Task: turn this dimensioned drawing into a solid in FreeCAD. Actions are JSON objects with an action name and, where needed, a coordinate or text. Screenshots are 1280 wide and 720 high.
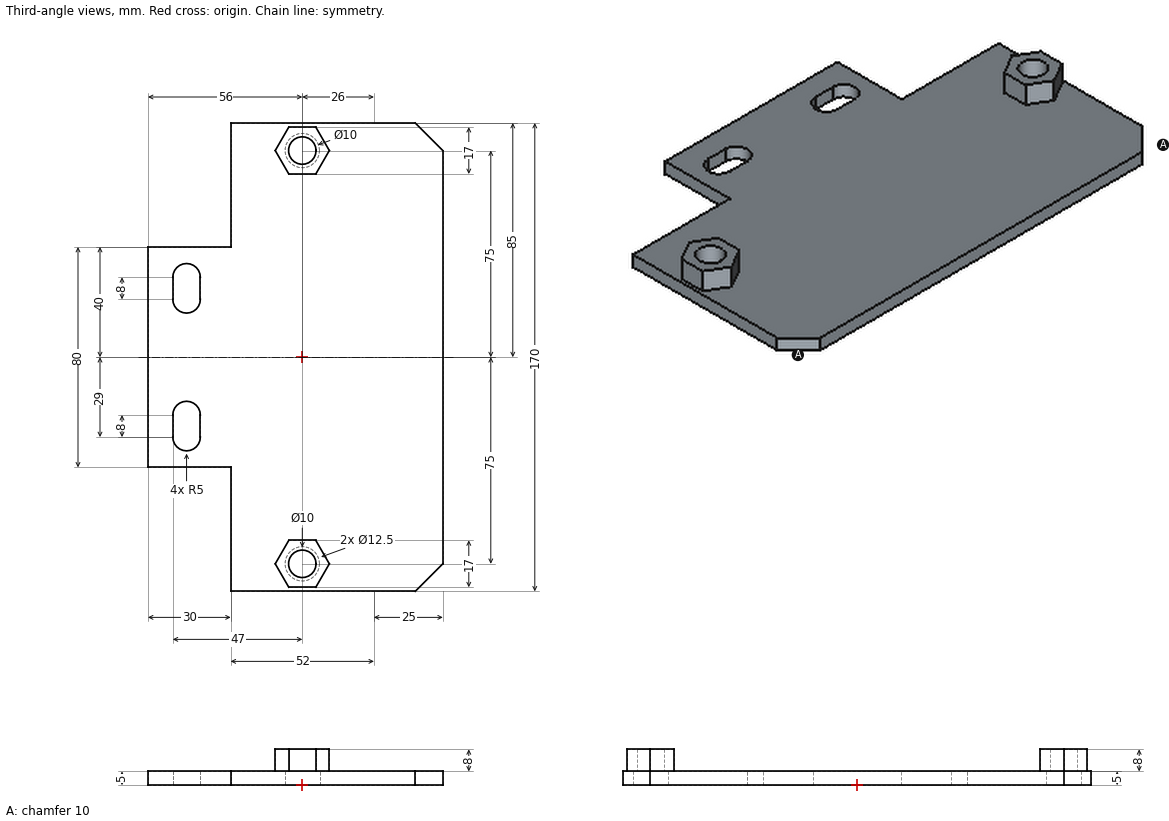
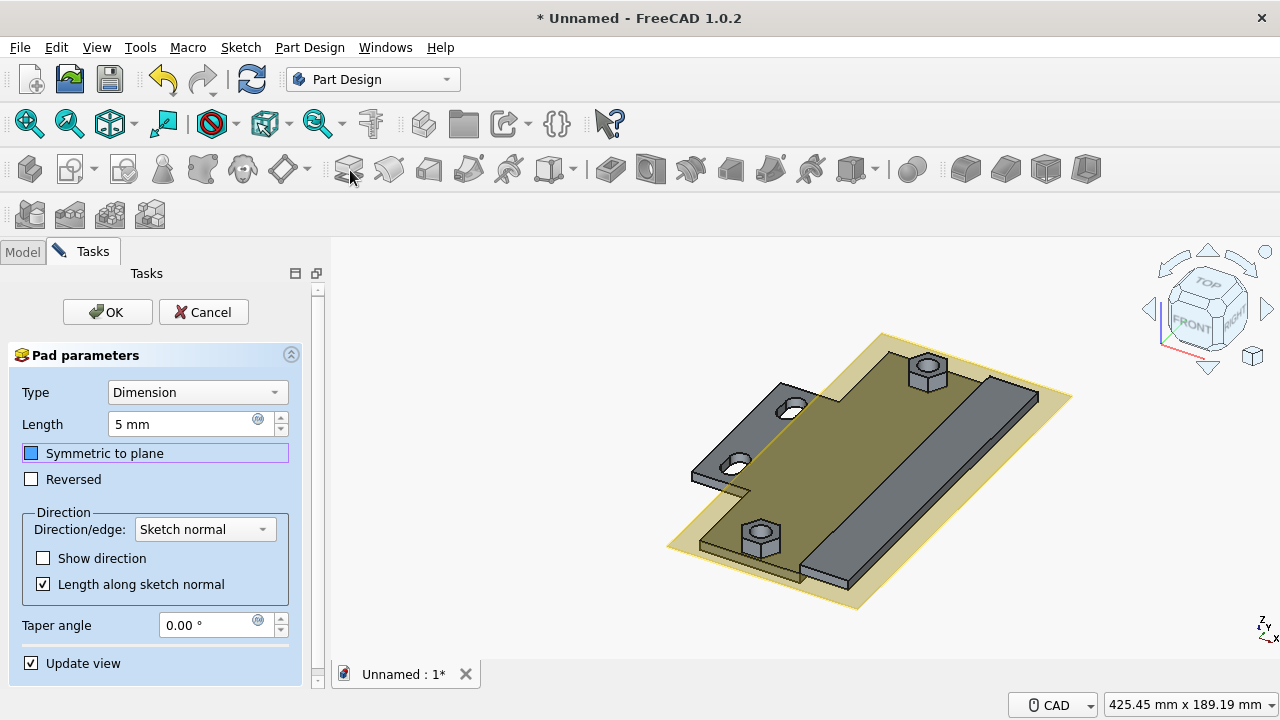
{"action": "left_click", "coordinate": [30, 479]}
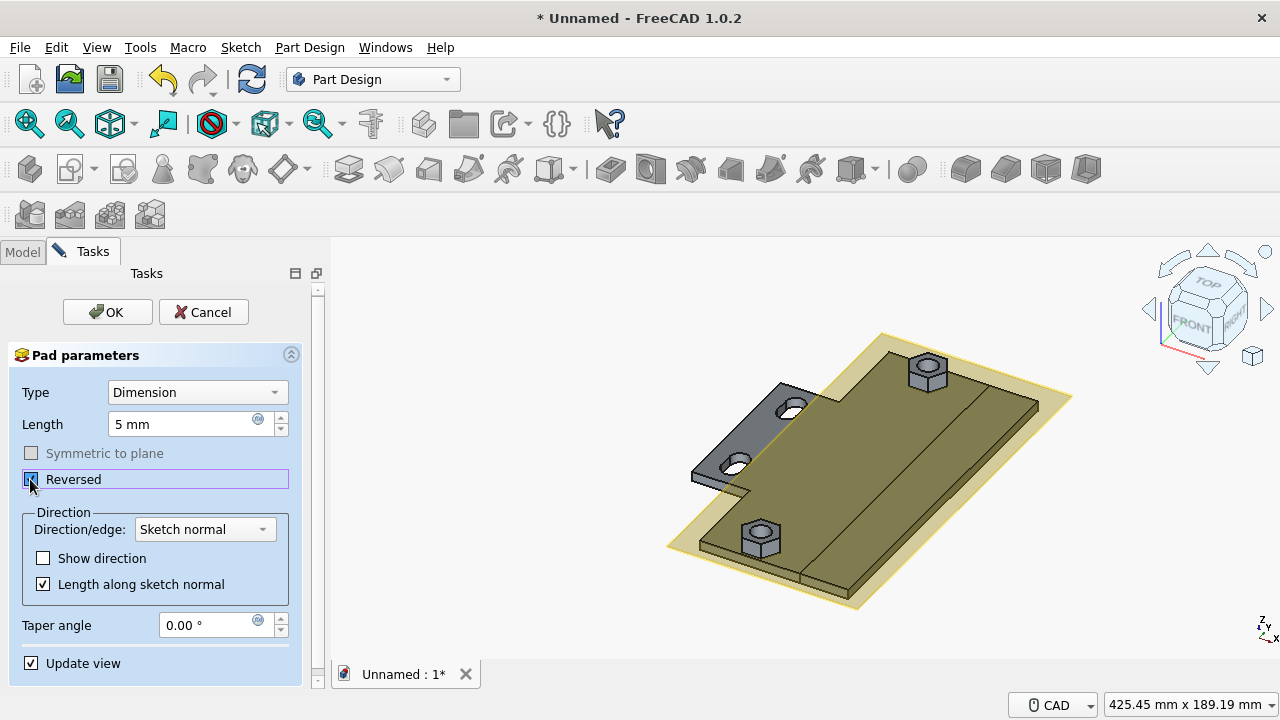
{"action": "left_click", "coordinate": [108, 312]}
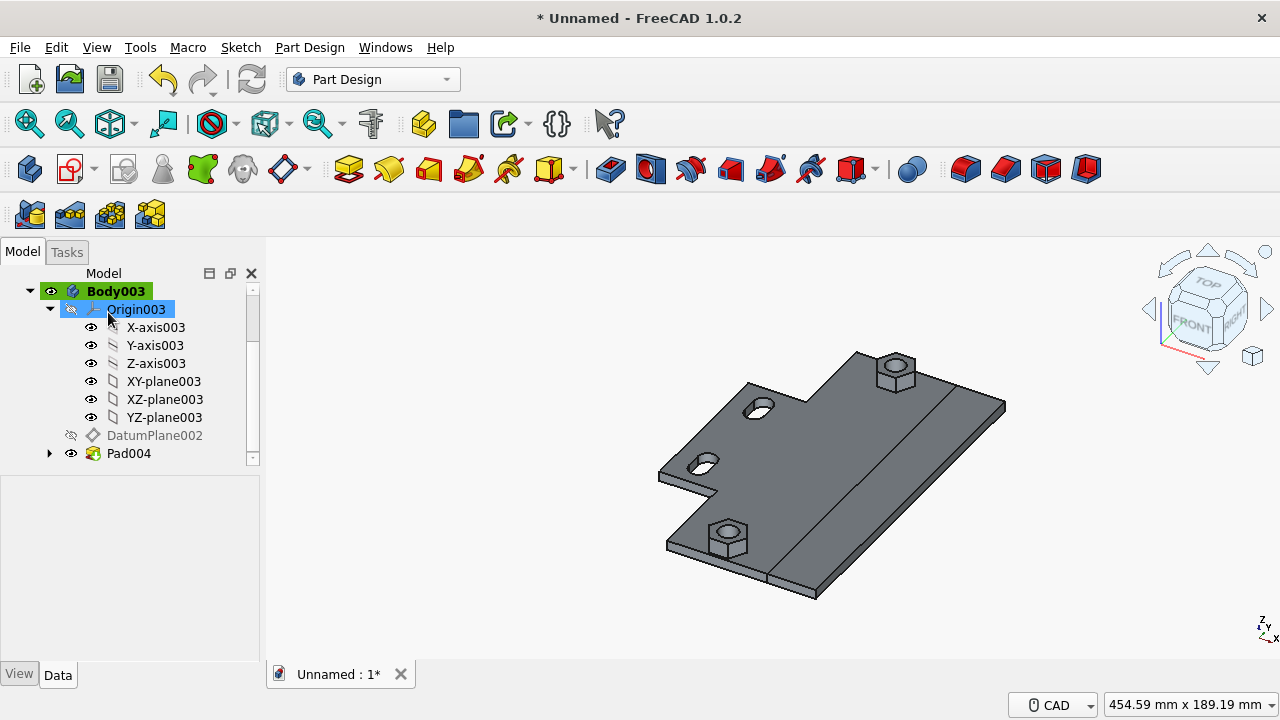
{"action": "scroll", "coordinate": [120, 377], "scroll_direction": "down", "scroll_amount": 3}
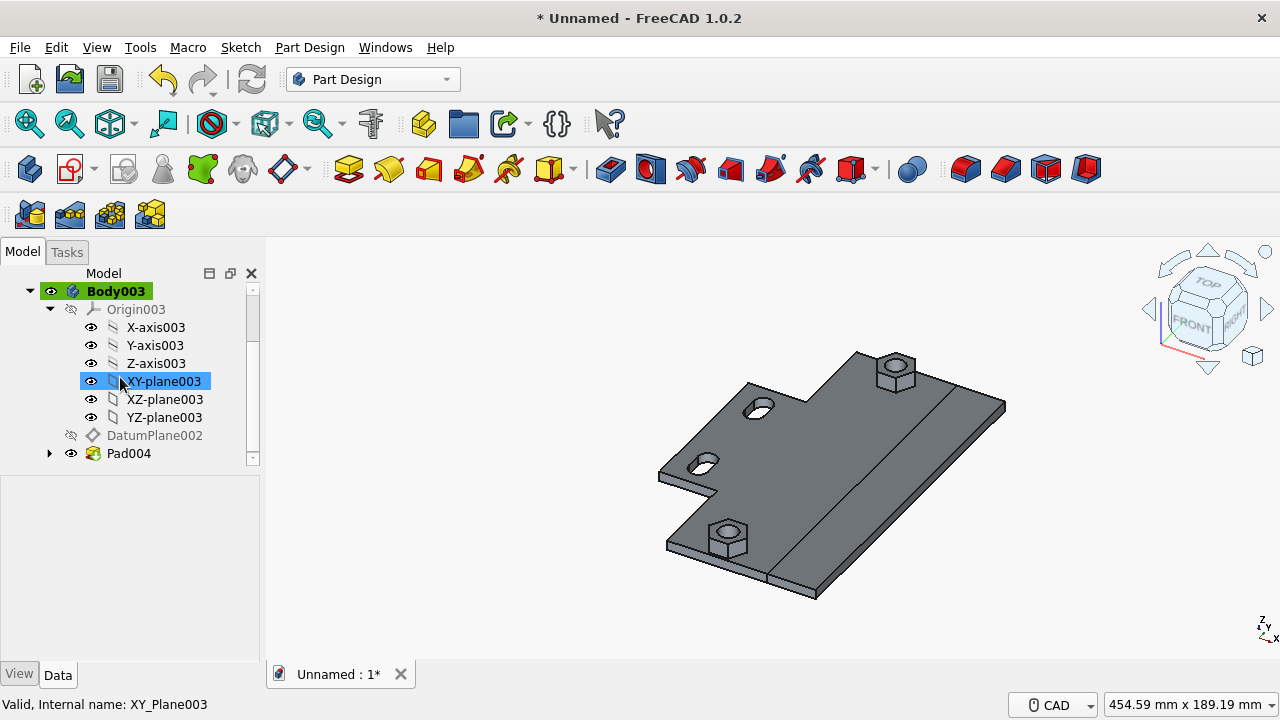
{"action": "scroll", "coordinate": [120, 377], "scroll_direction": "up", "scroll_amount": 15}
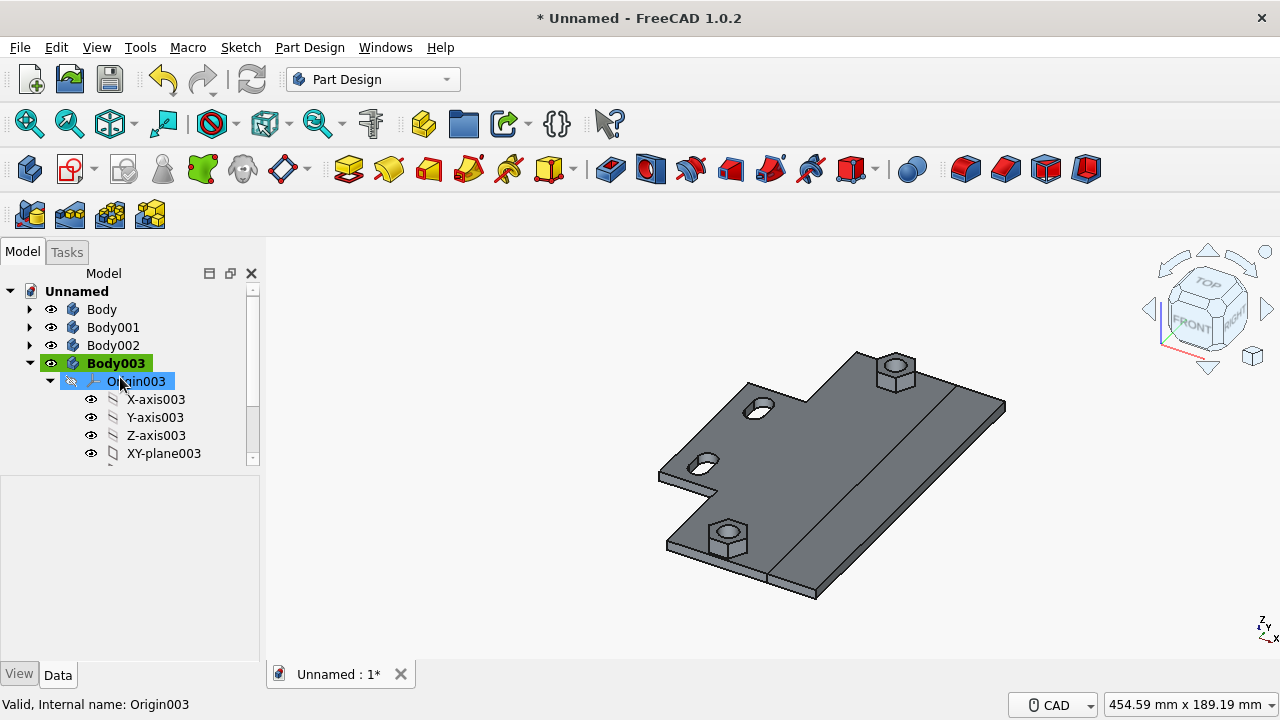
{"action": "double_click", "coordinate": [96, 309]}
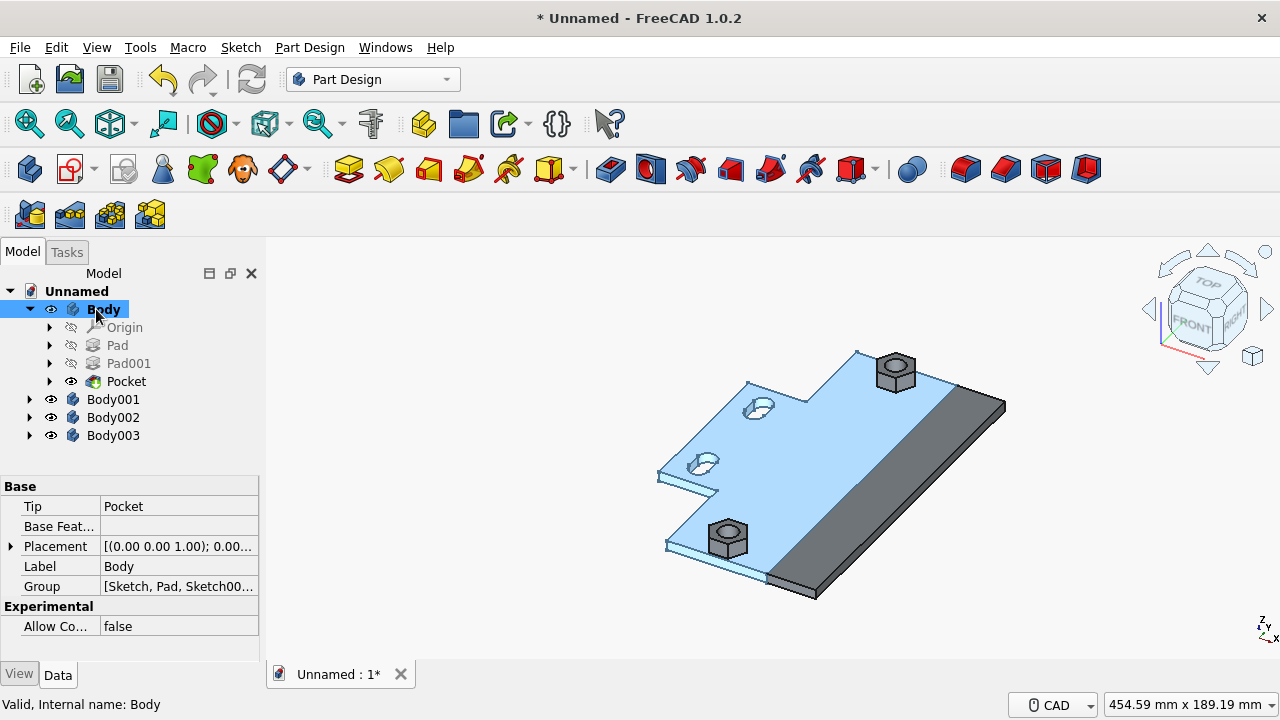
{"action": "left_click", "coordinate": [96, 435]}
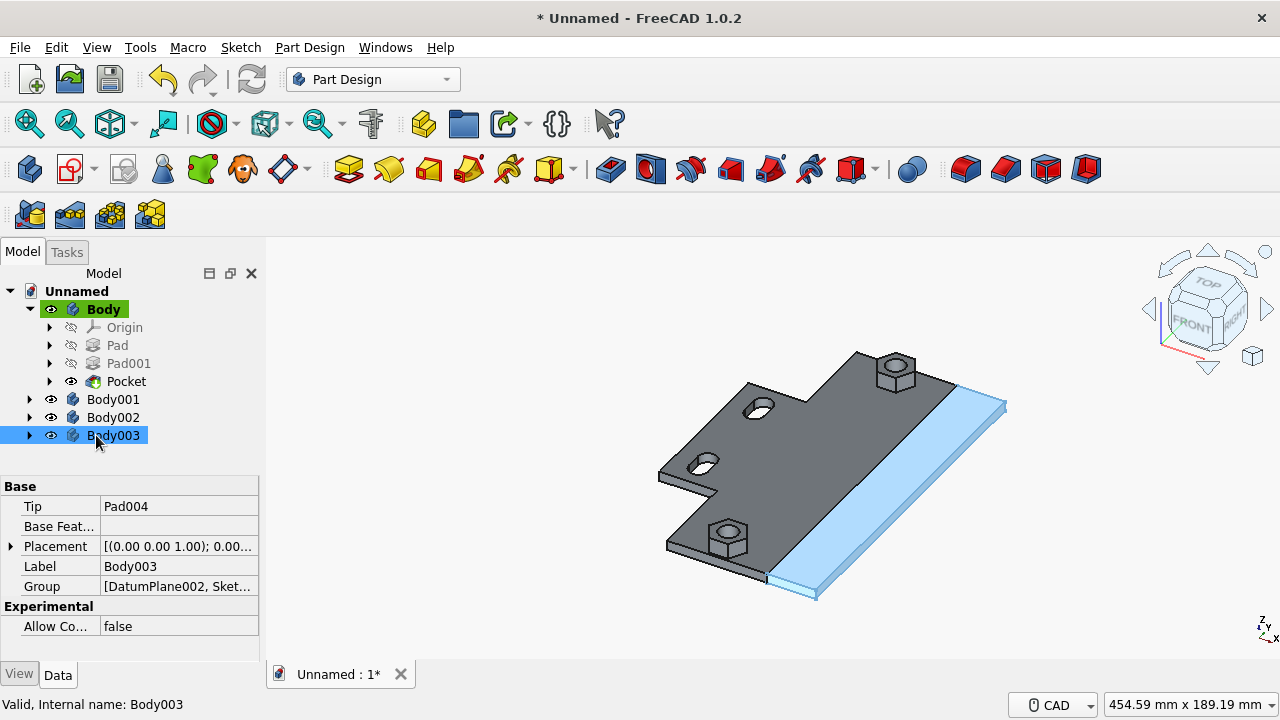
{"action": "left_click", "coordinate": [914, 170]}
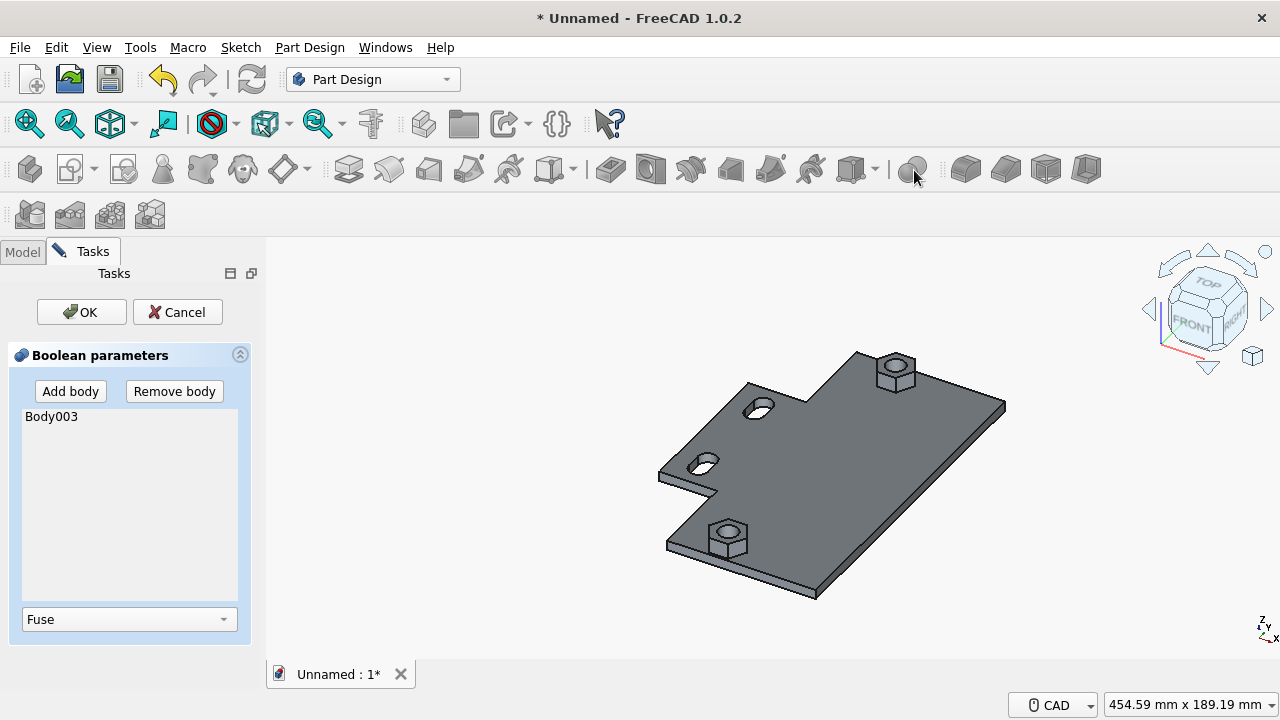
{"action": "left_click", "coordinate": [82, 312]}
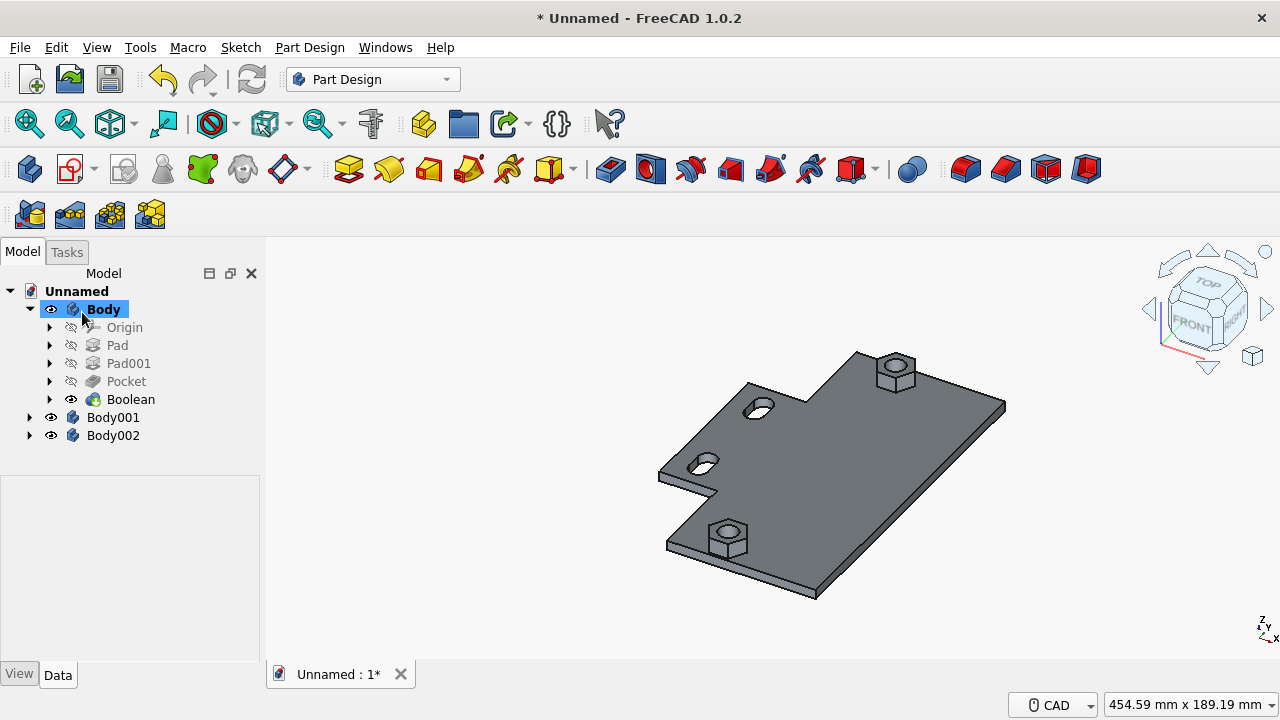
{"action": "left_click", "coordinate": [816, 595]}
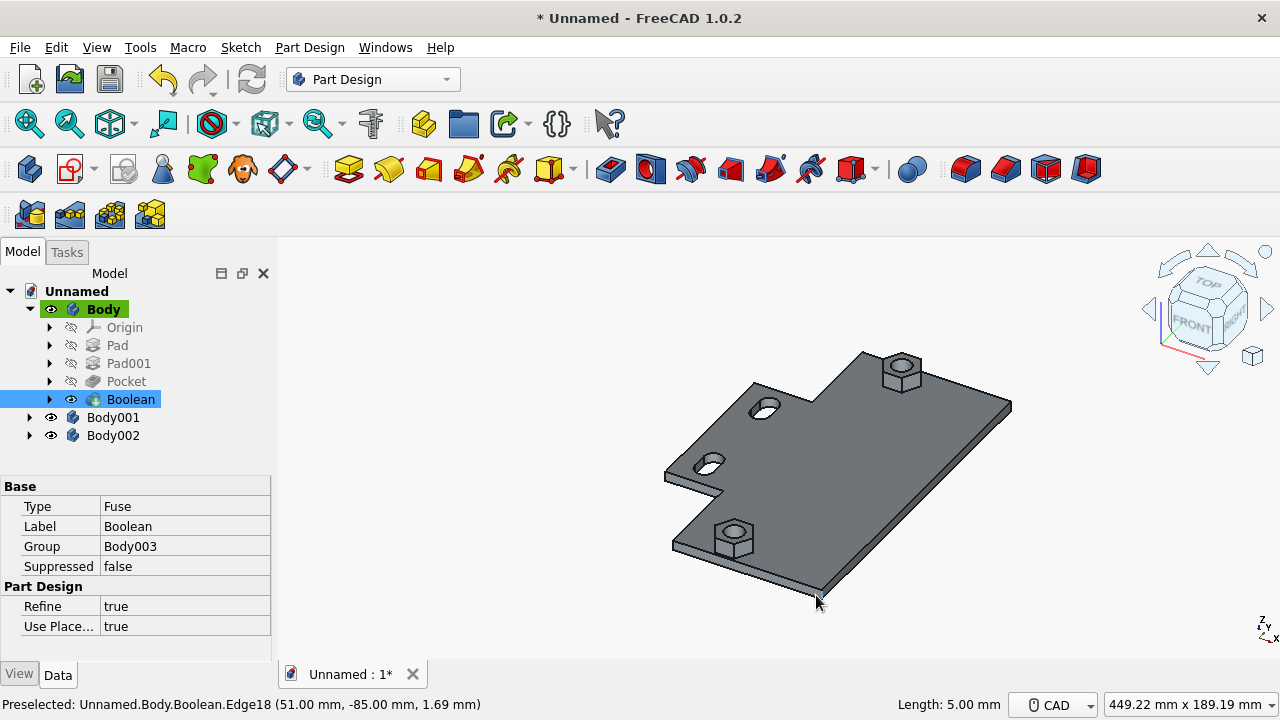
{"action": "scroll", "coordinate": [1011, 405], "scroll_direction": "up", "scroll_amount": 7}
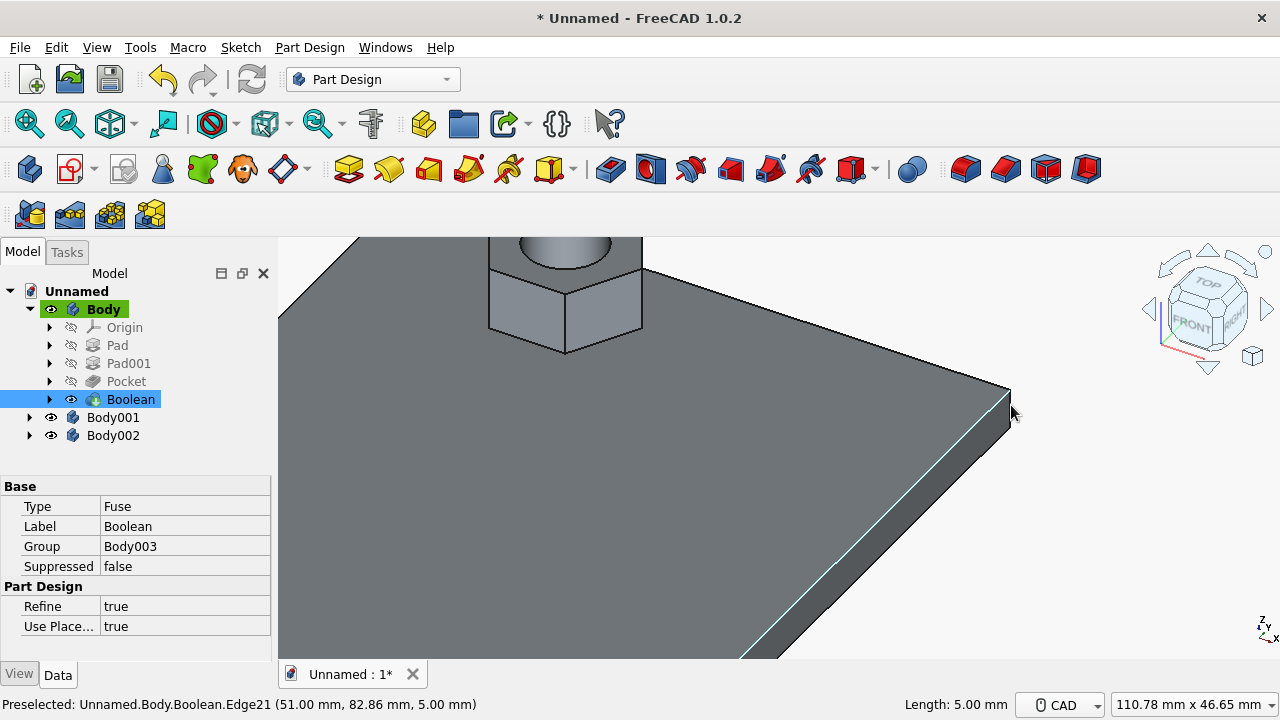
{"action": "left_click", "coordinate": [30, 124]}